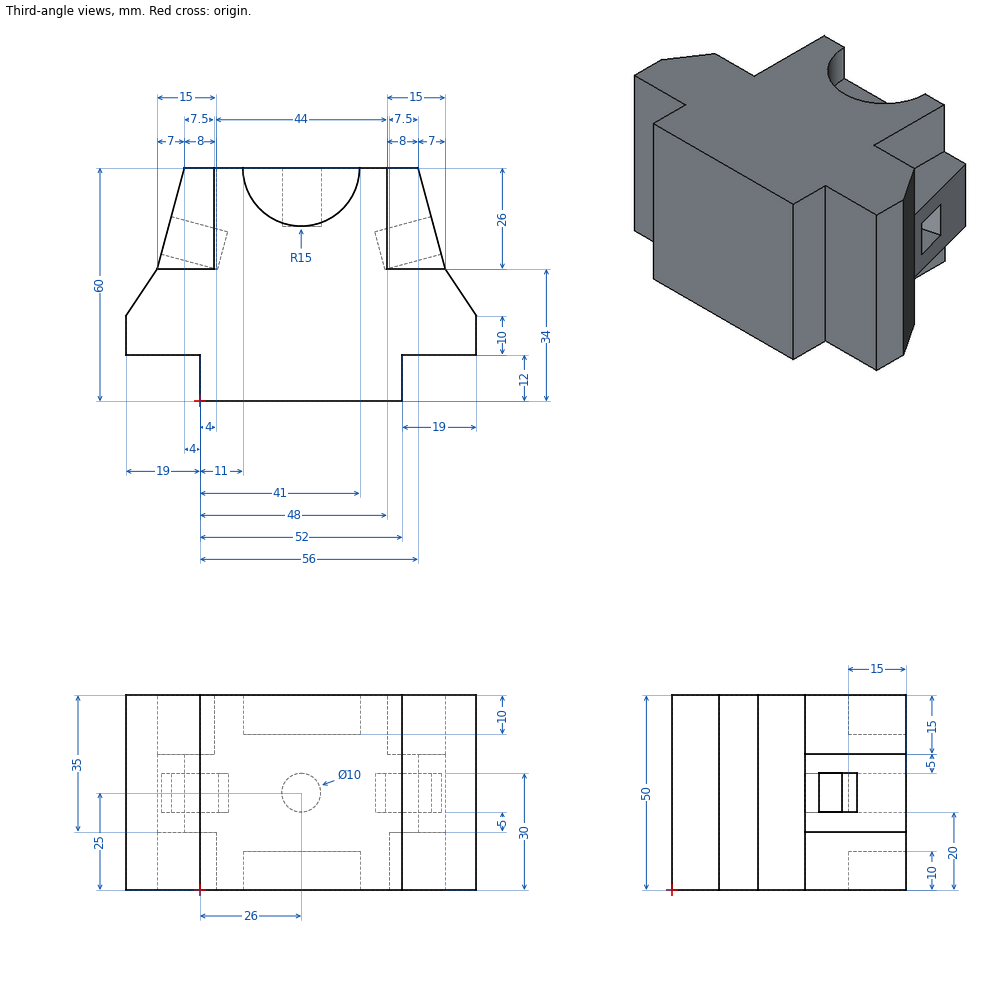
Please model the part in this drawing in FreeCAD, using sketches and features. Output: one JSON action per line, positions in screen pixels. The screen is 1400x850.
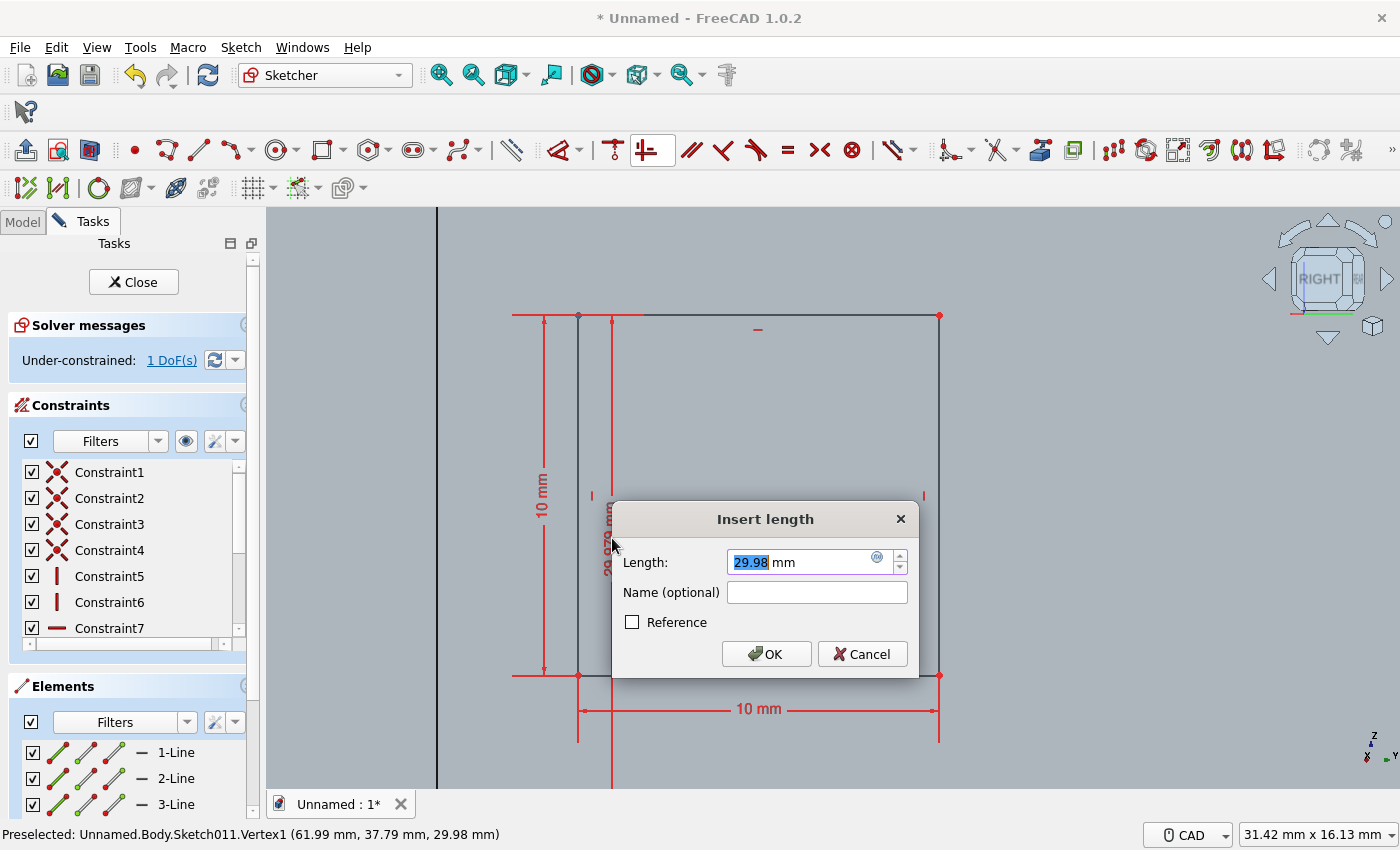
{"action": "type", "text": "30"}
{"action": "key", "text": "Return"}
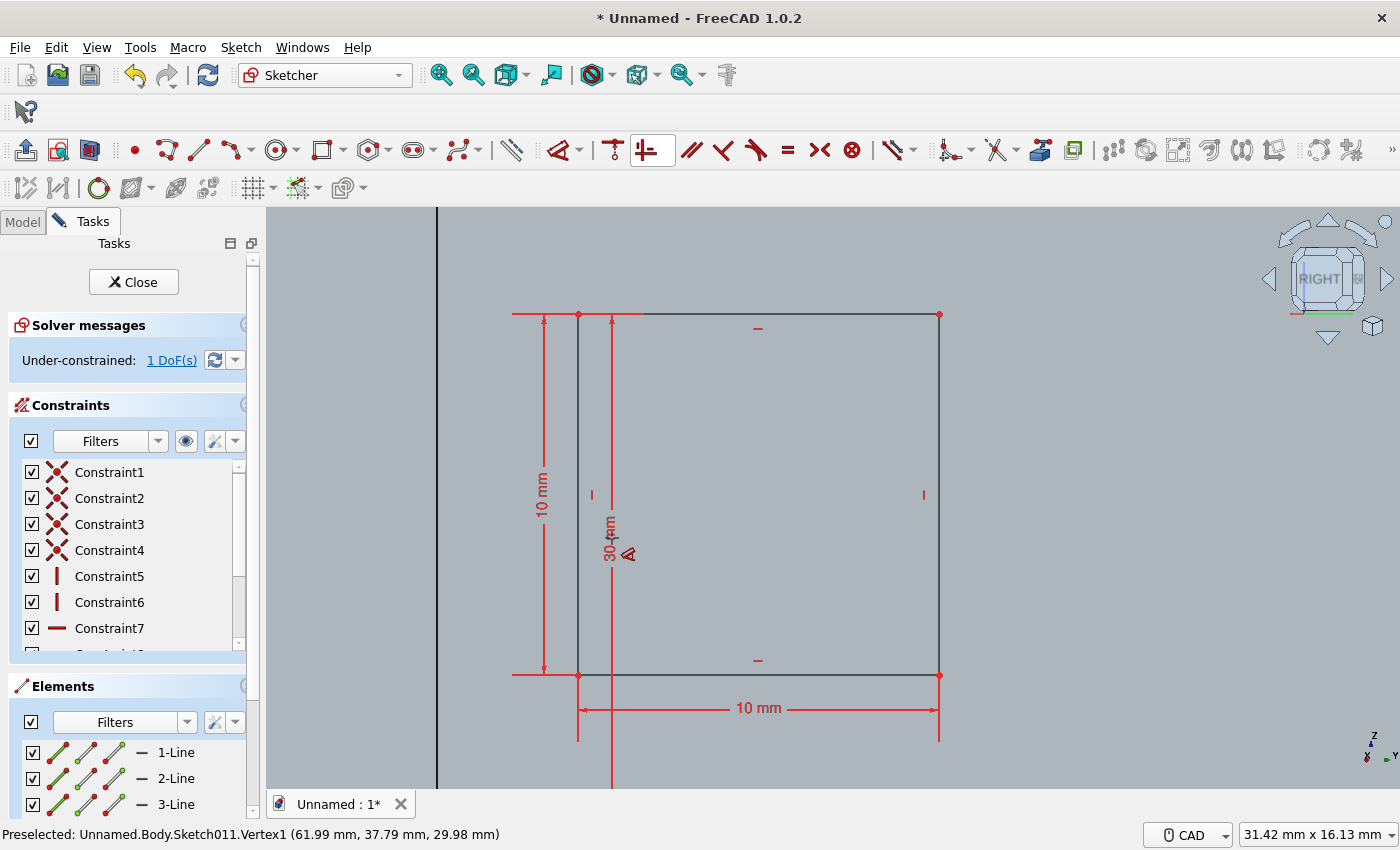
{"action": "left_click", "coordinate": [578, 314]}
{"action": "left_click", "coordinate": [436, 280]}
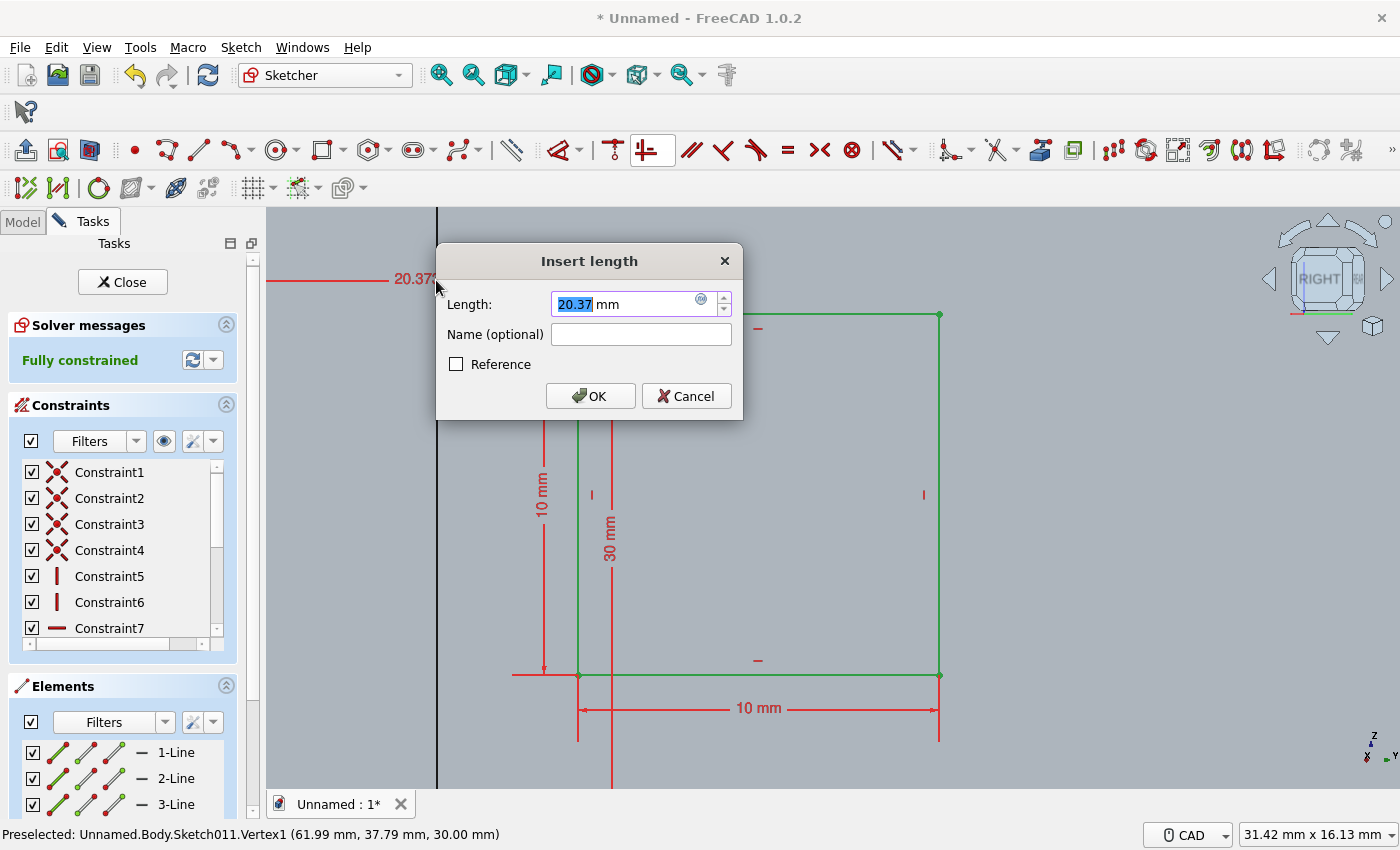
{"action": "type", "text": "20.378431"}
{"action": "key", "text": "Return"}
{"action": "key", "text": "Escape"}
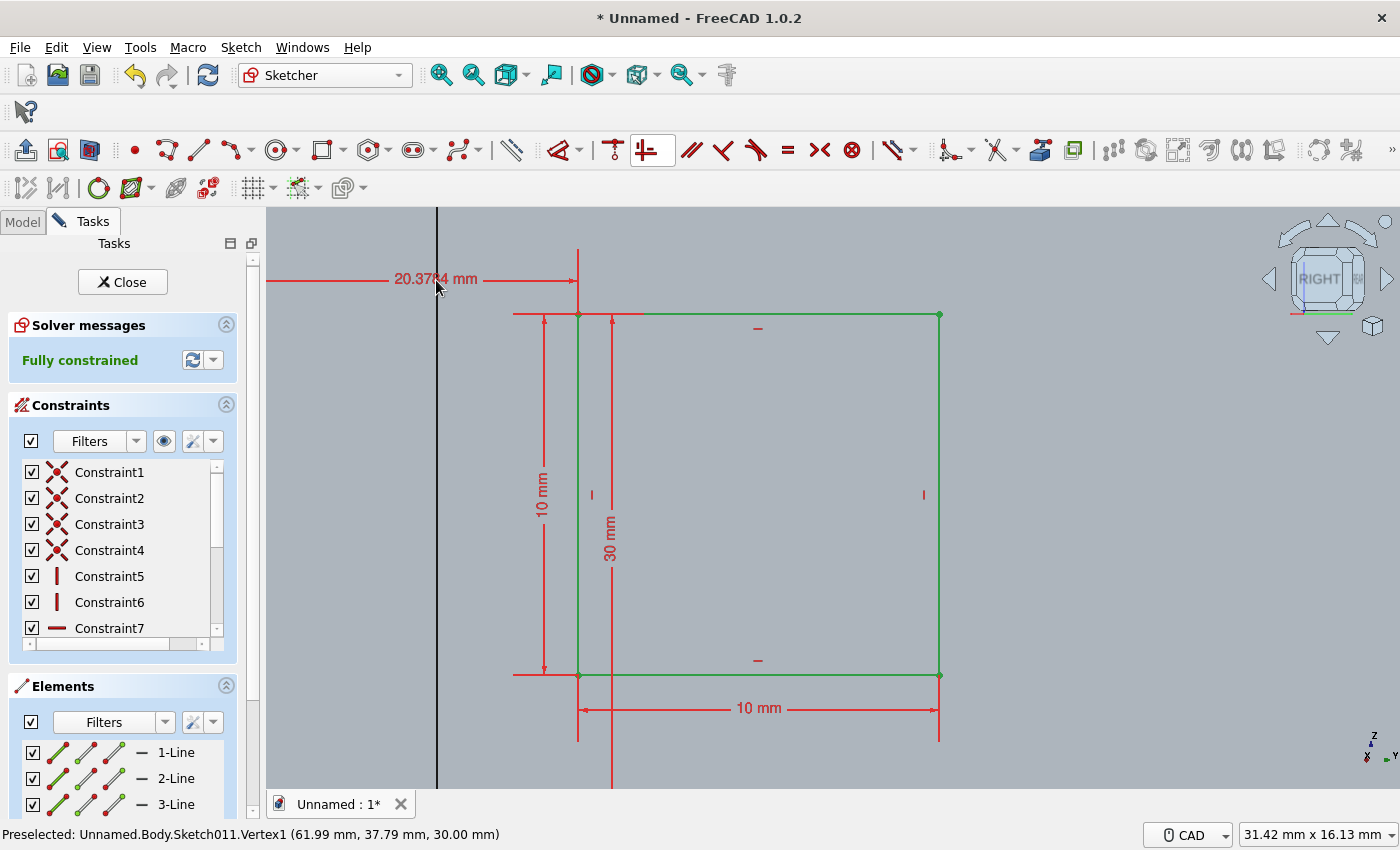
{"action": "left_click", "coordinate": [123, 282]}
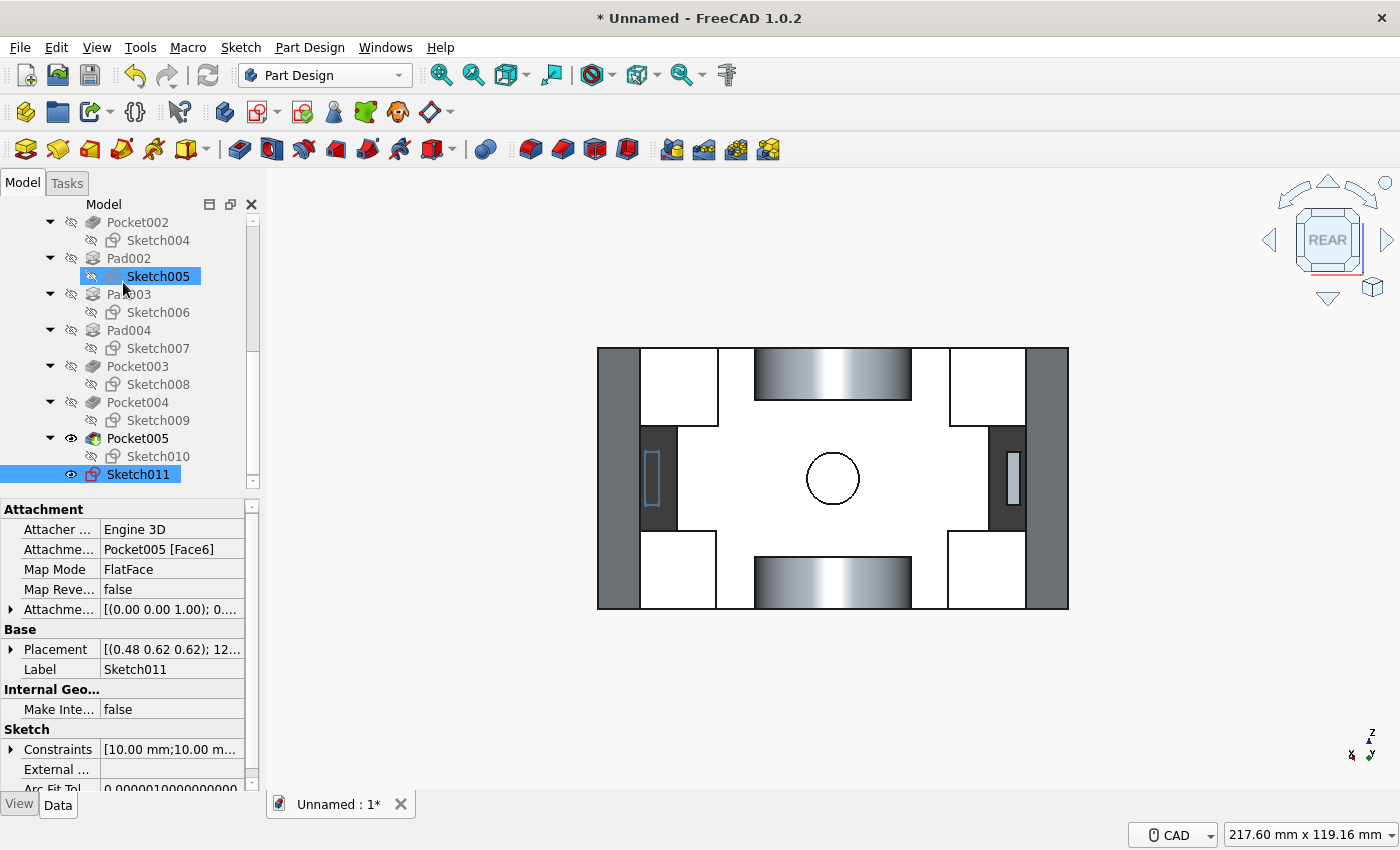
{"action": "left_click", "coordinate": [240, 150]}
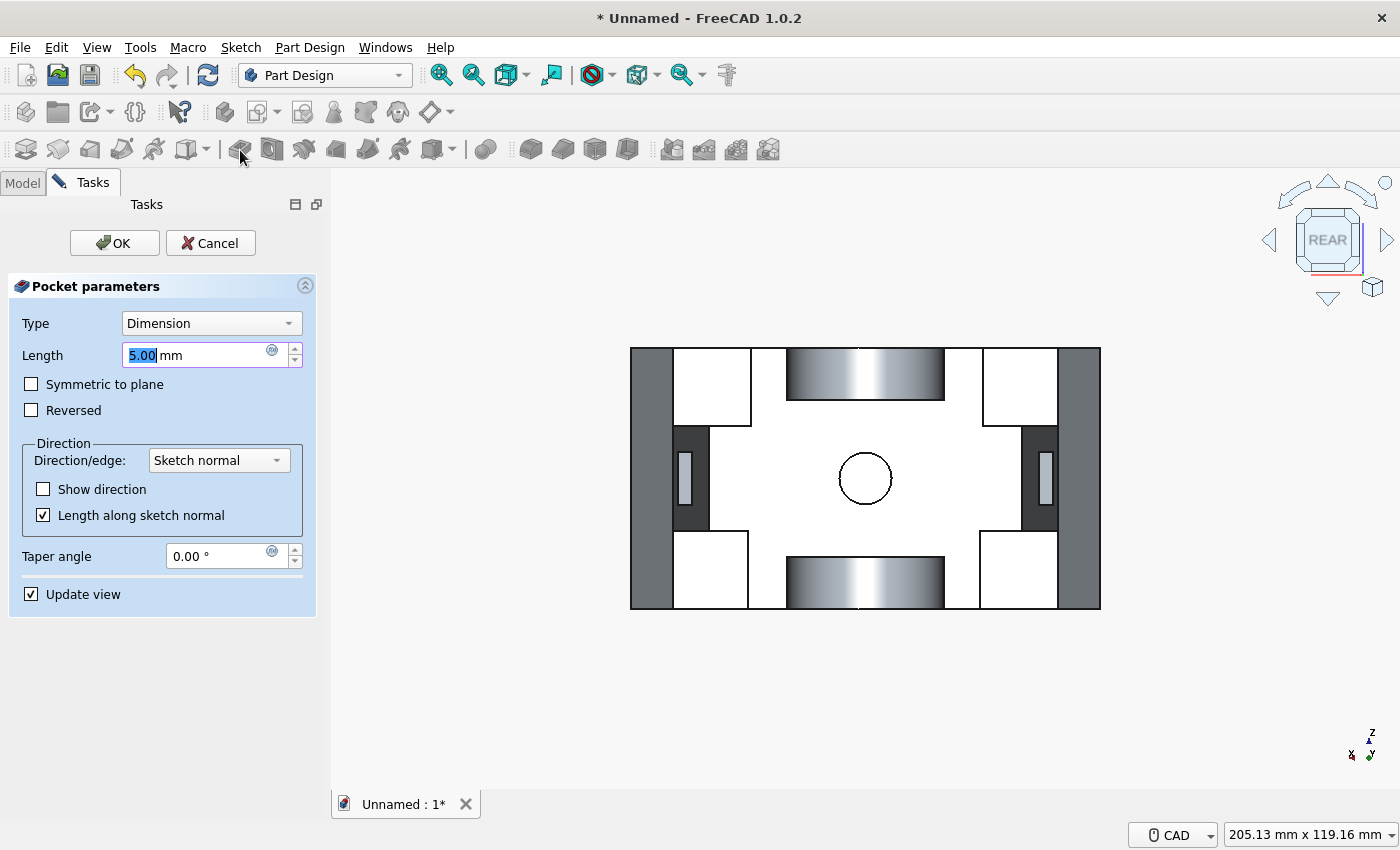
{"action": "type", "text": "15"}
{"action": "key", "text": "Tab"}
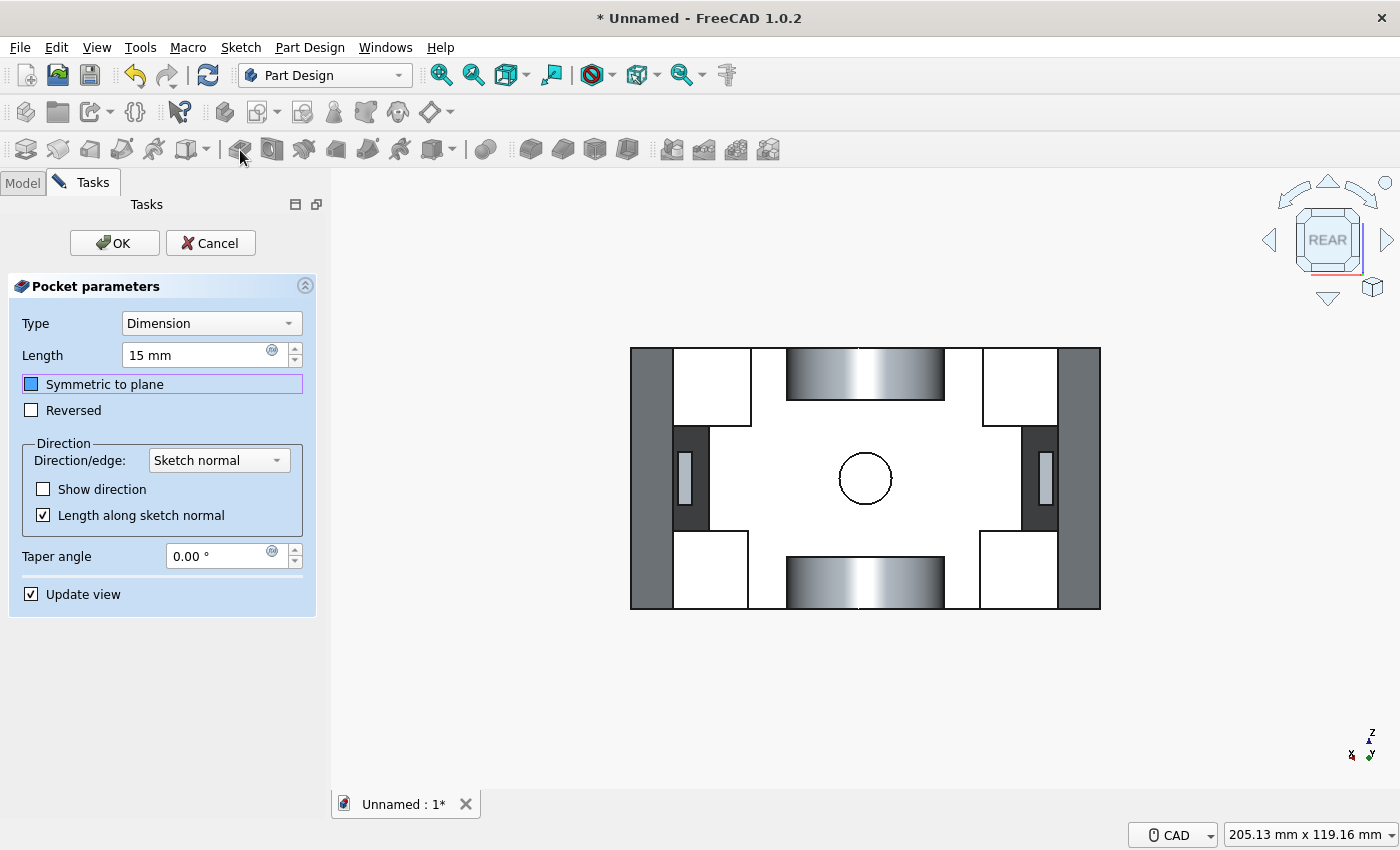
{"action": "left_click", "coordinate": [115, 243]}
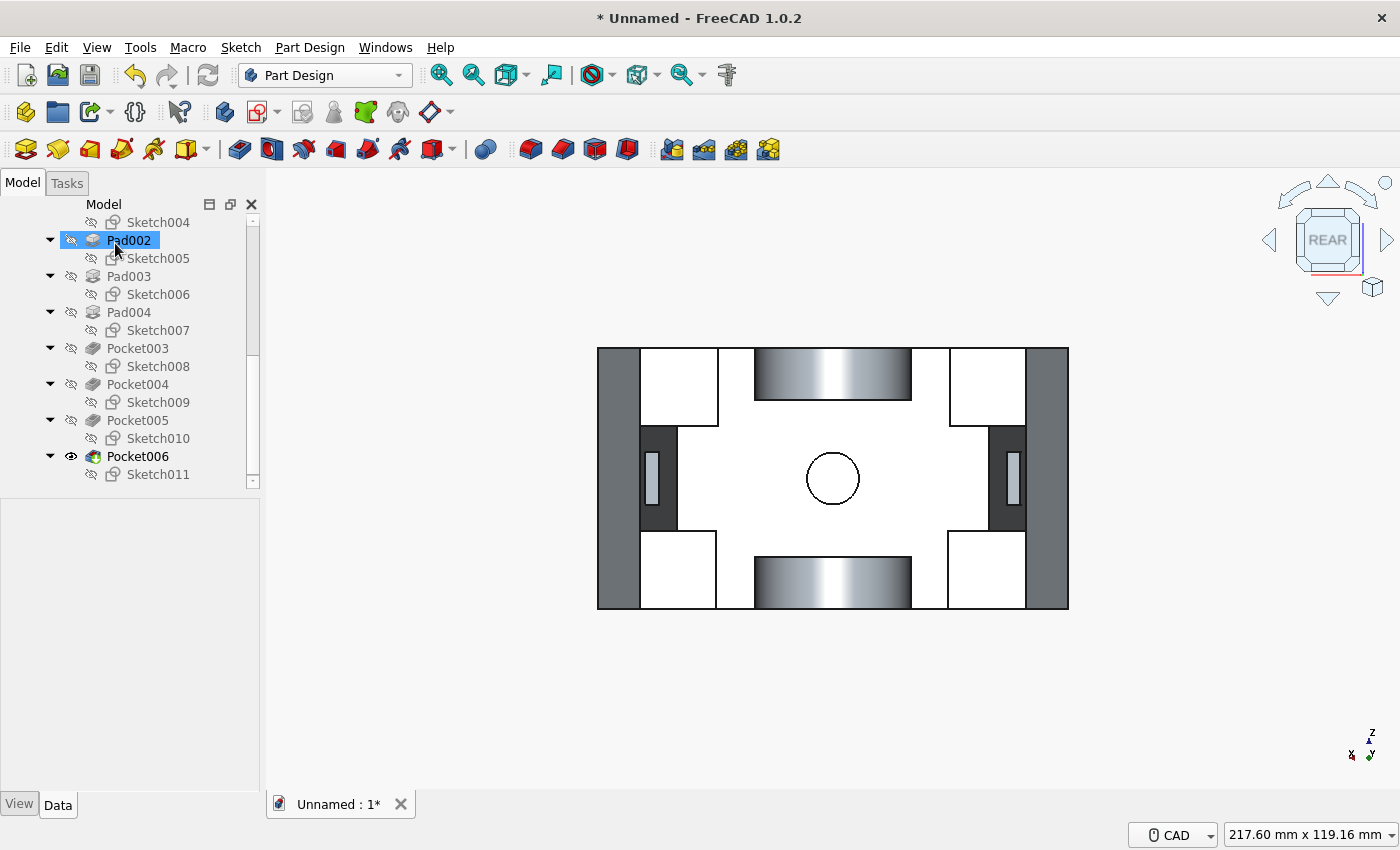
{"action": "key", "text": "0"}